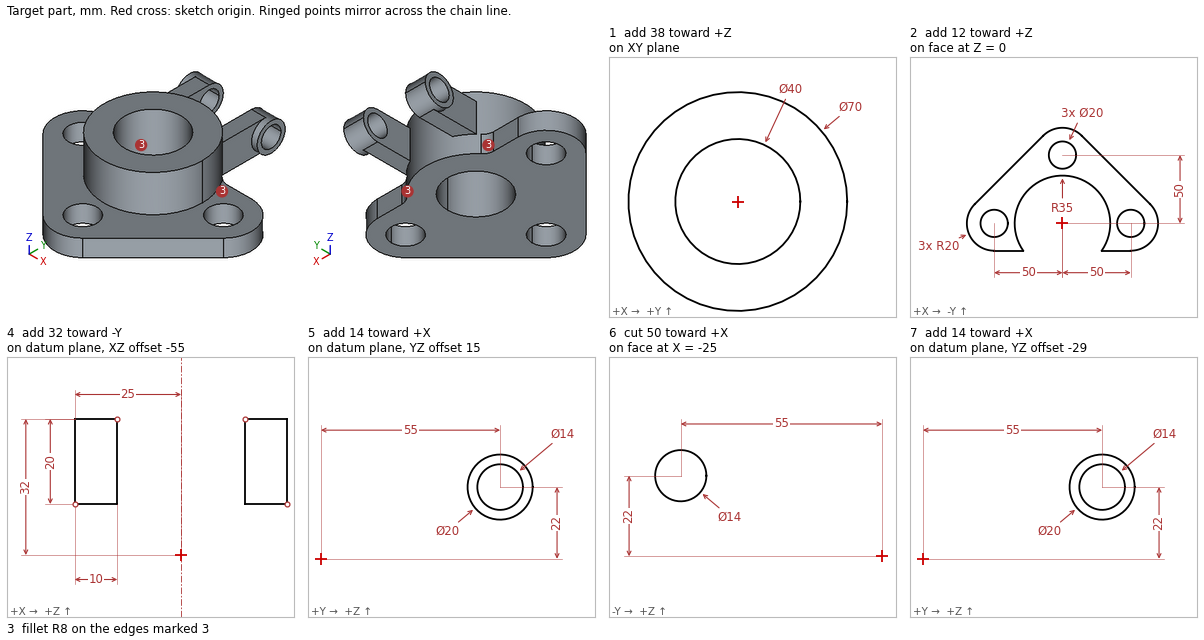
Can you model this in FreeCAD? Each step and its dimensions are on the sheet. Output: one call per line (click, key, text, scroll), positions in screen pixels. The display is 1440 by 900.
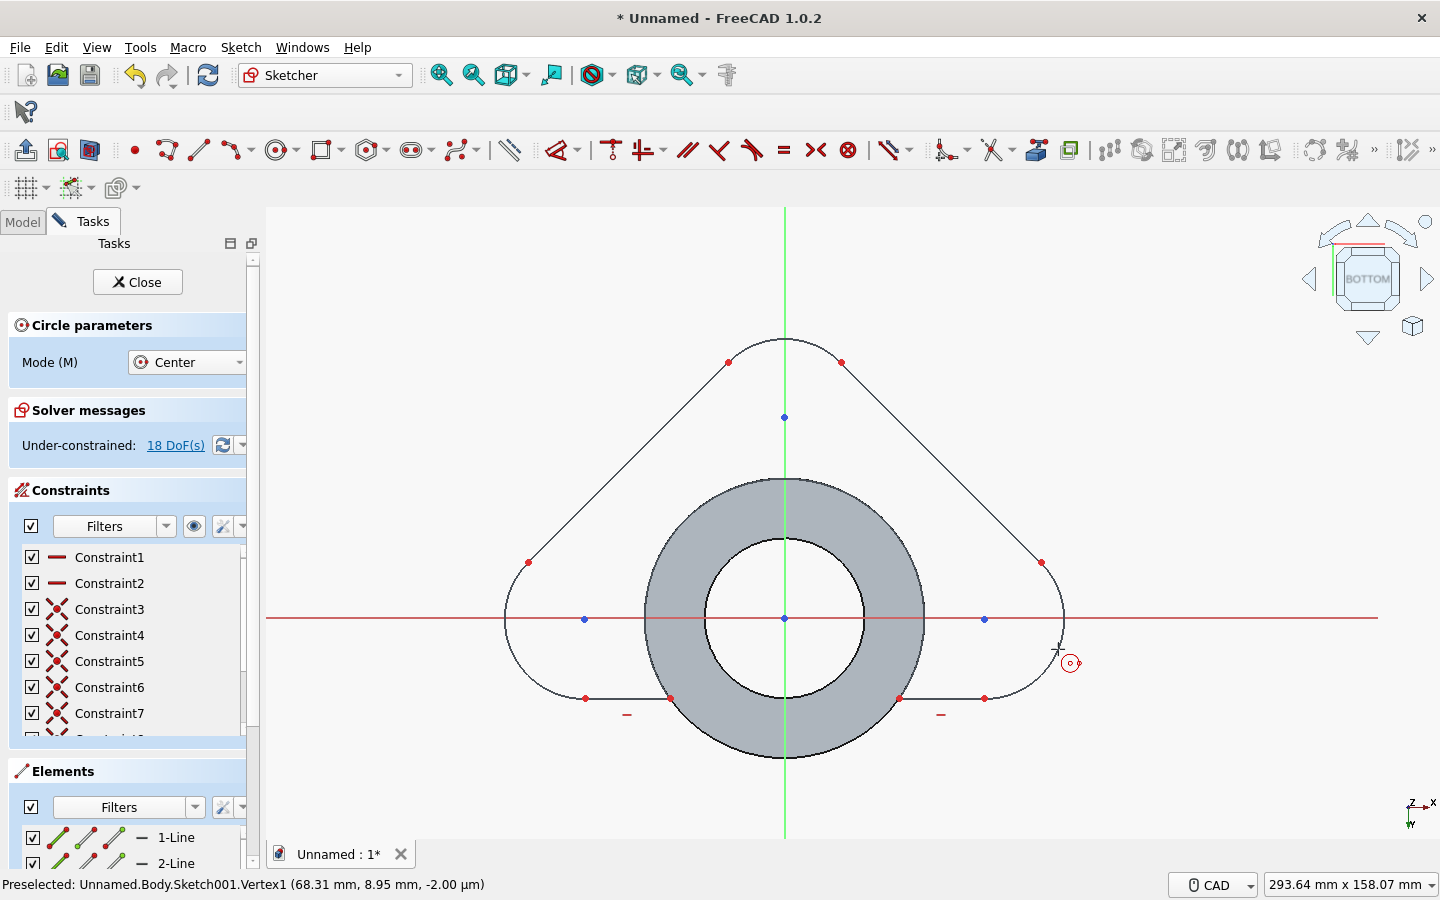
click(785, 418)
click(813, 390)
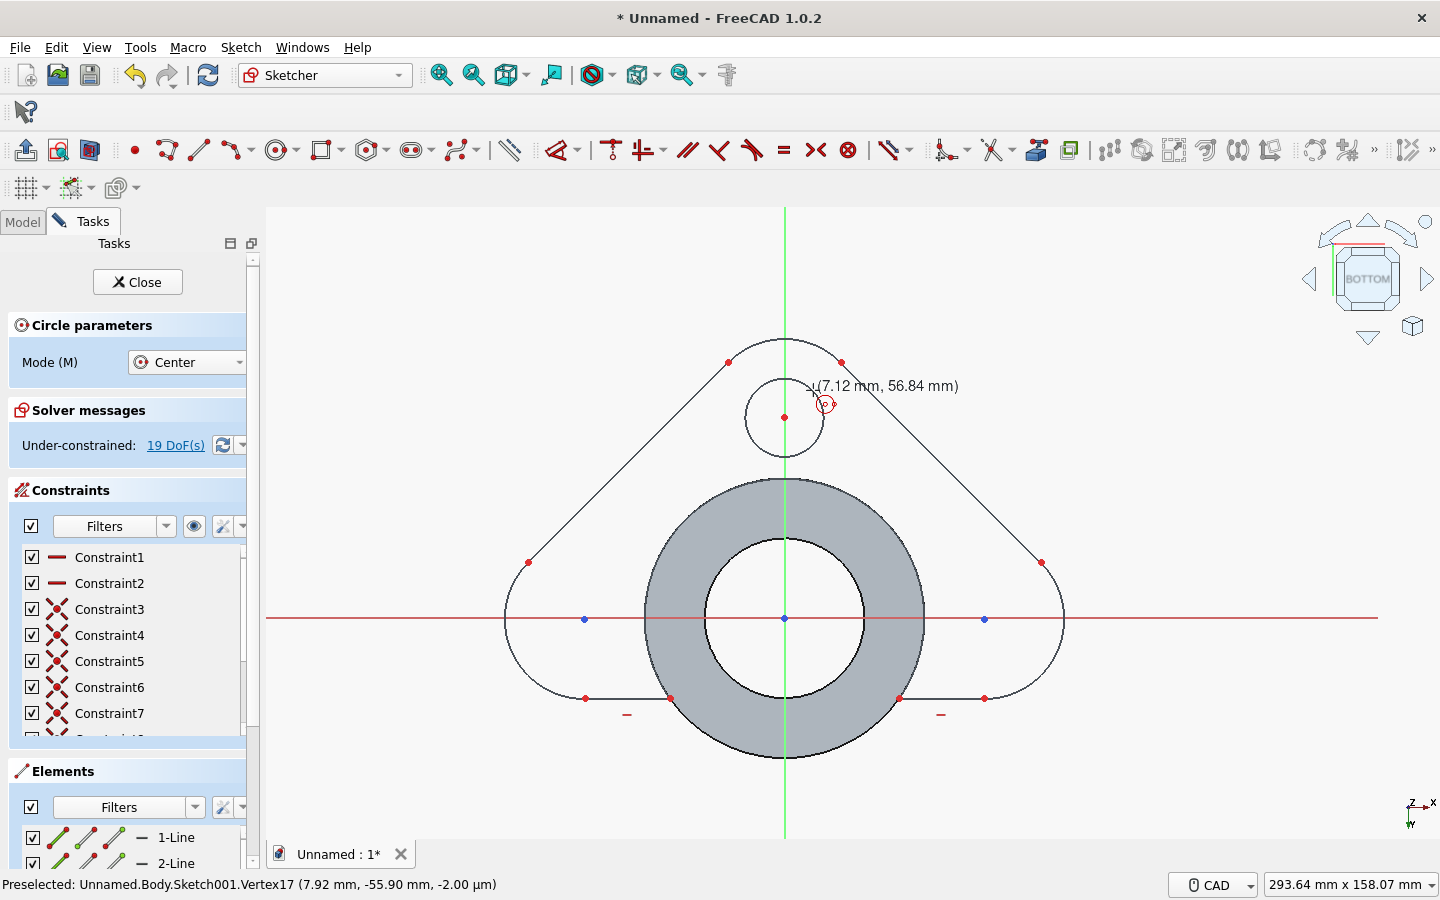
click(585, 618)
click(613, 590)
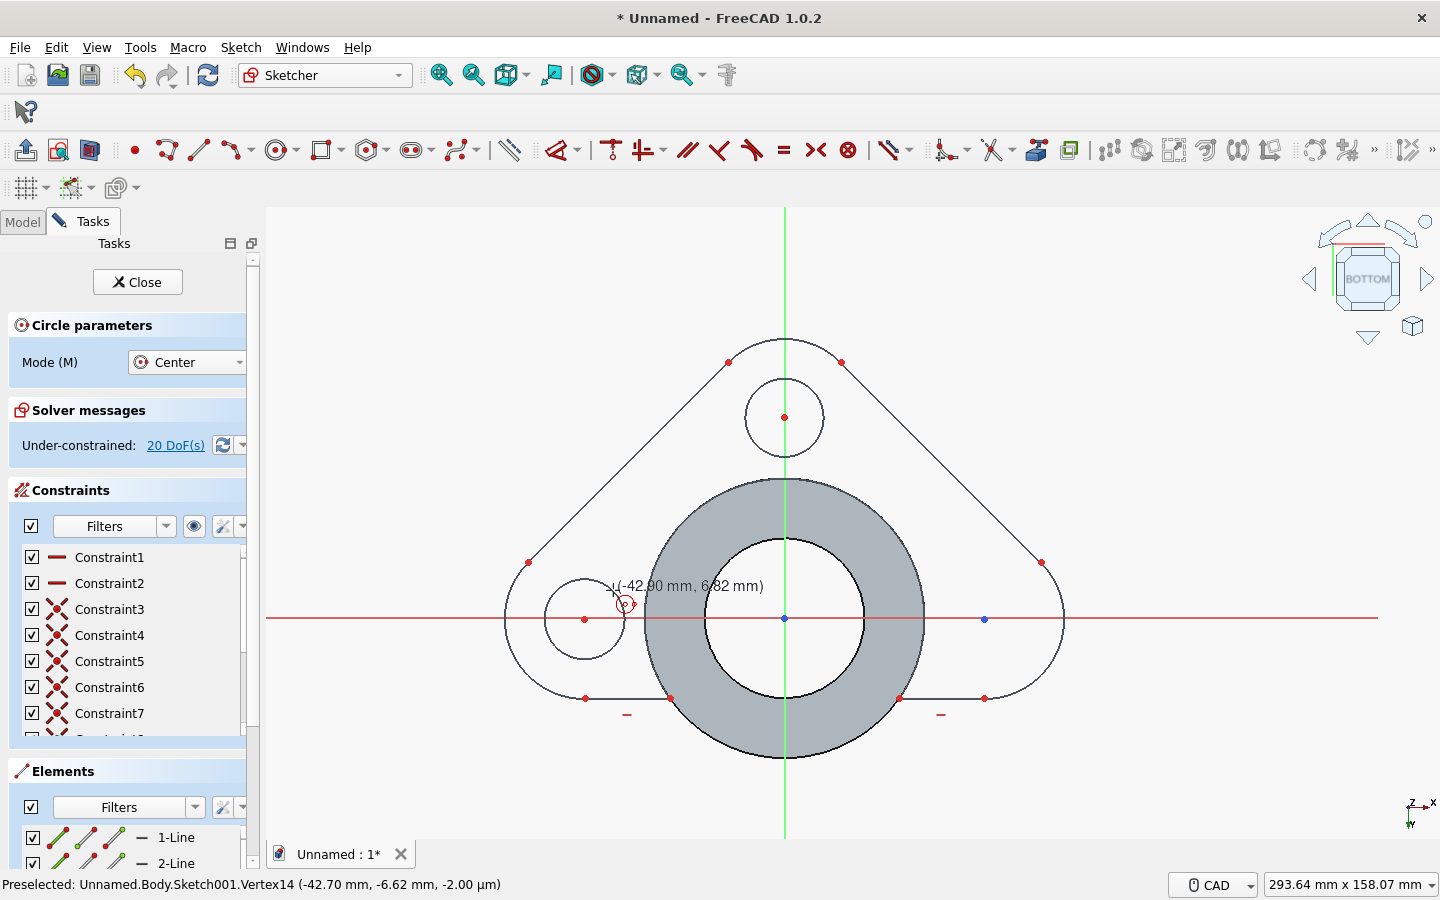
click(984, 618)
click(1013, 590)
key(Escape)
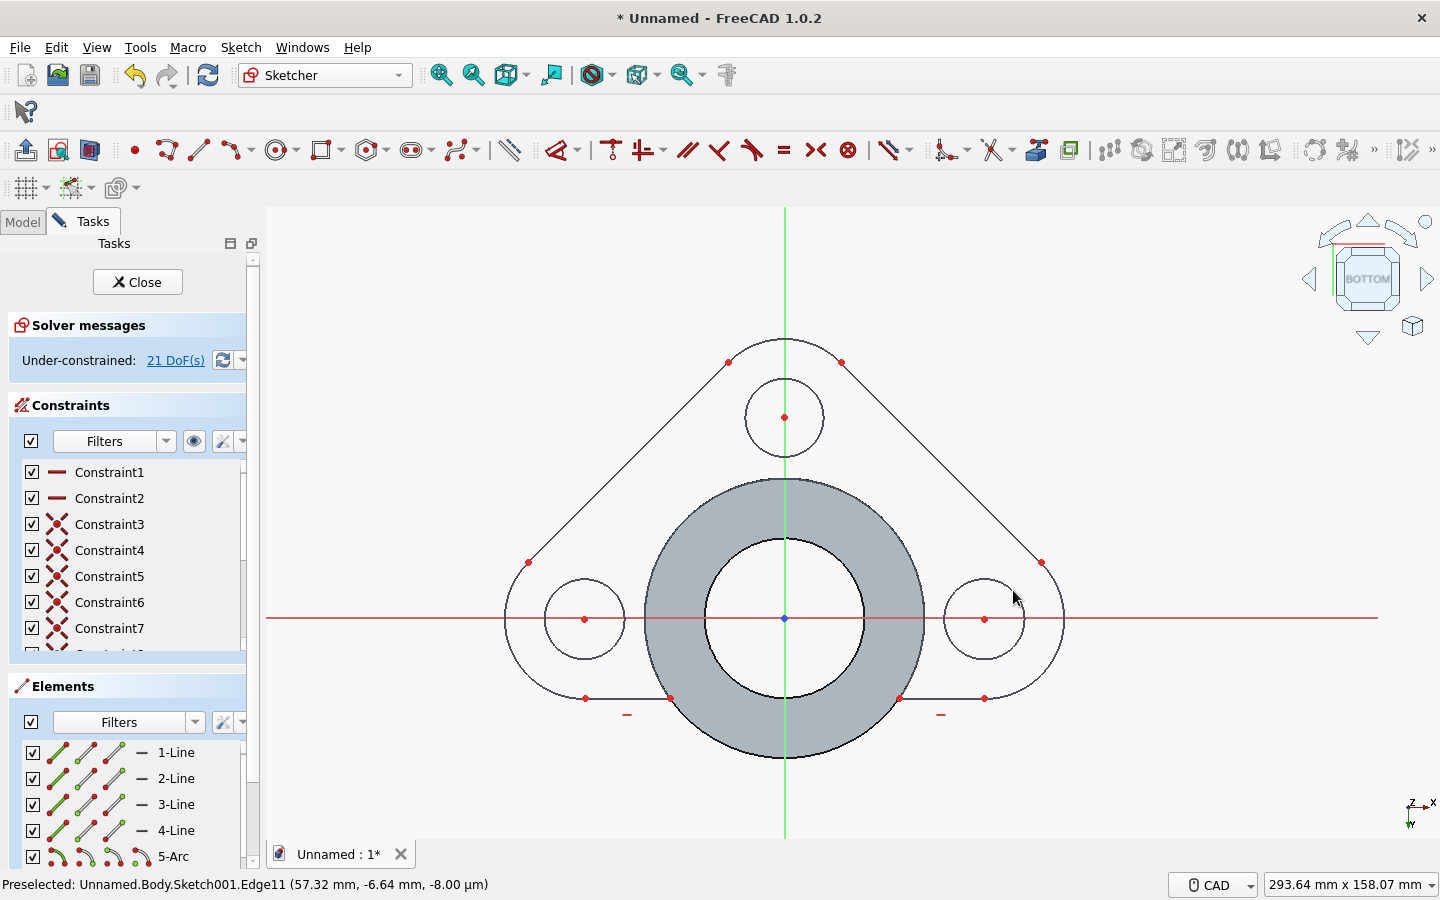
click(958, 699)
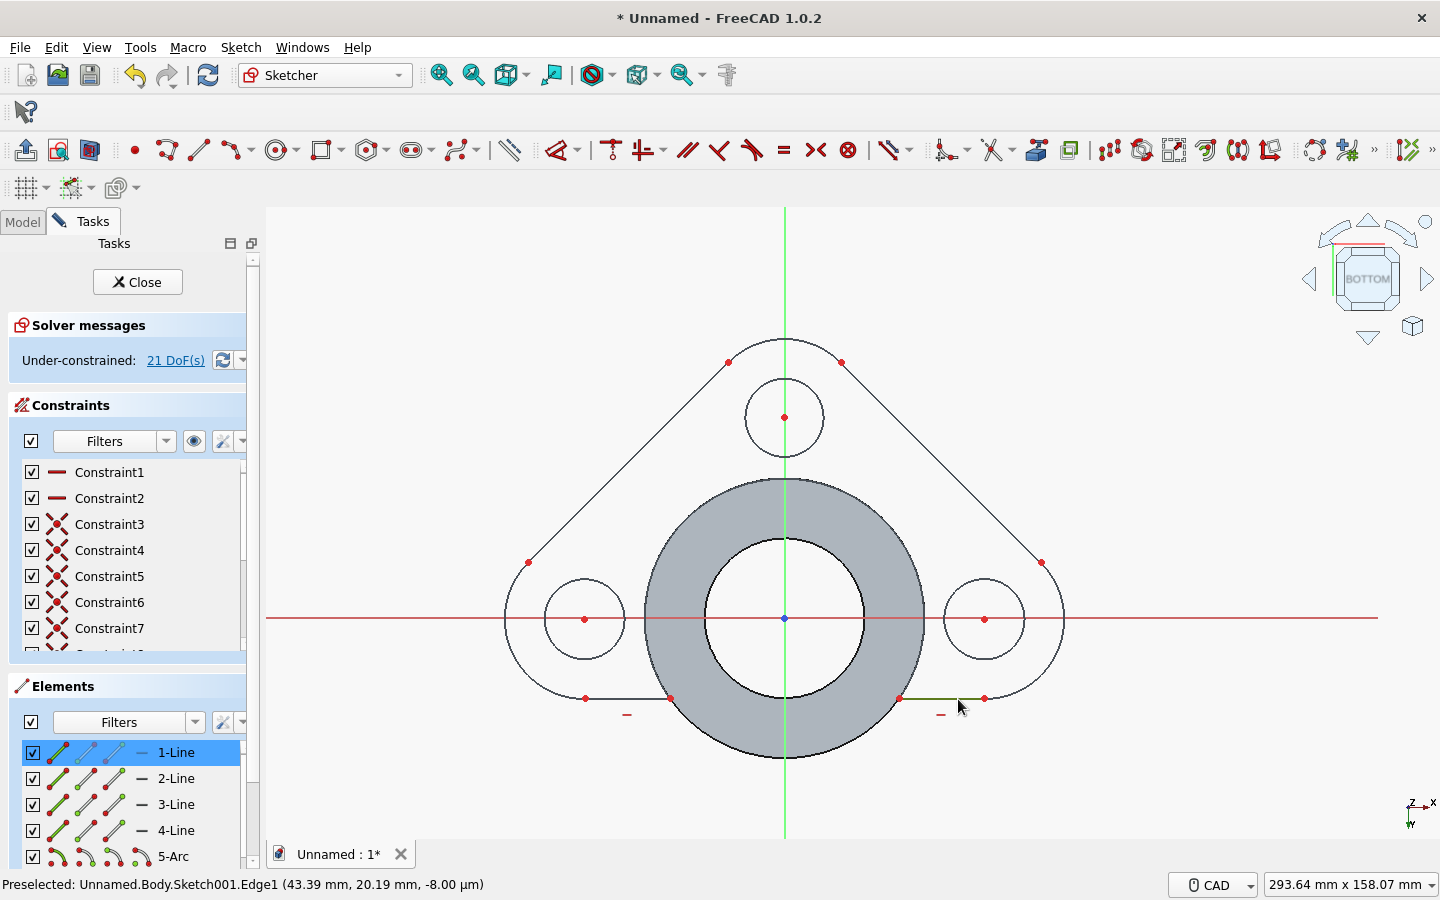
click(1036, 680)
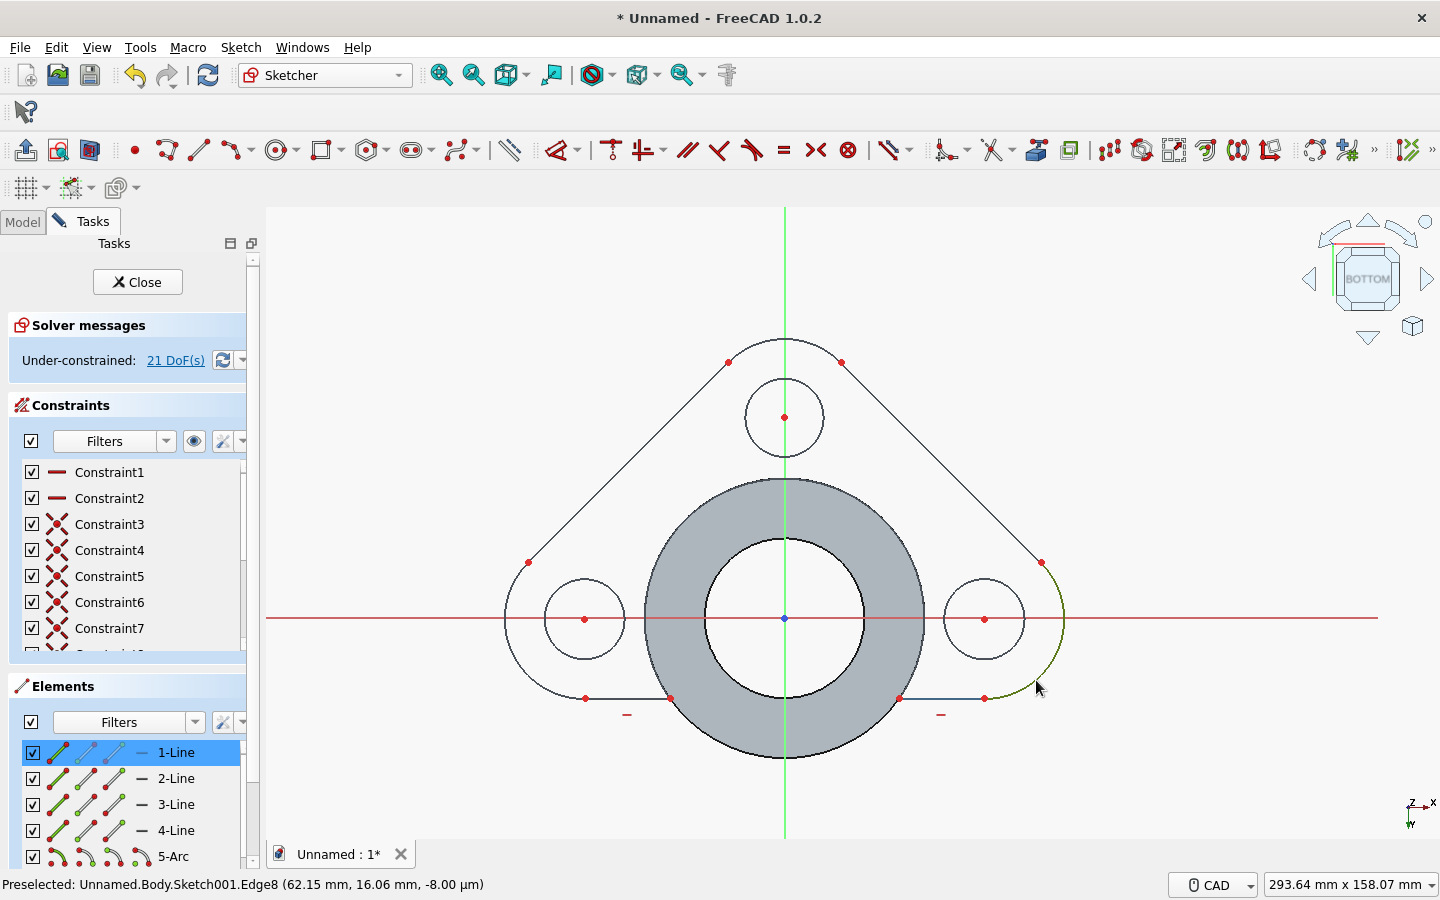
click(752, 150)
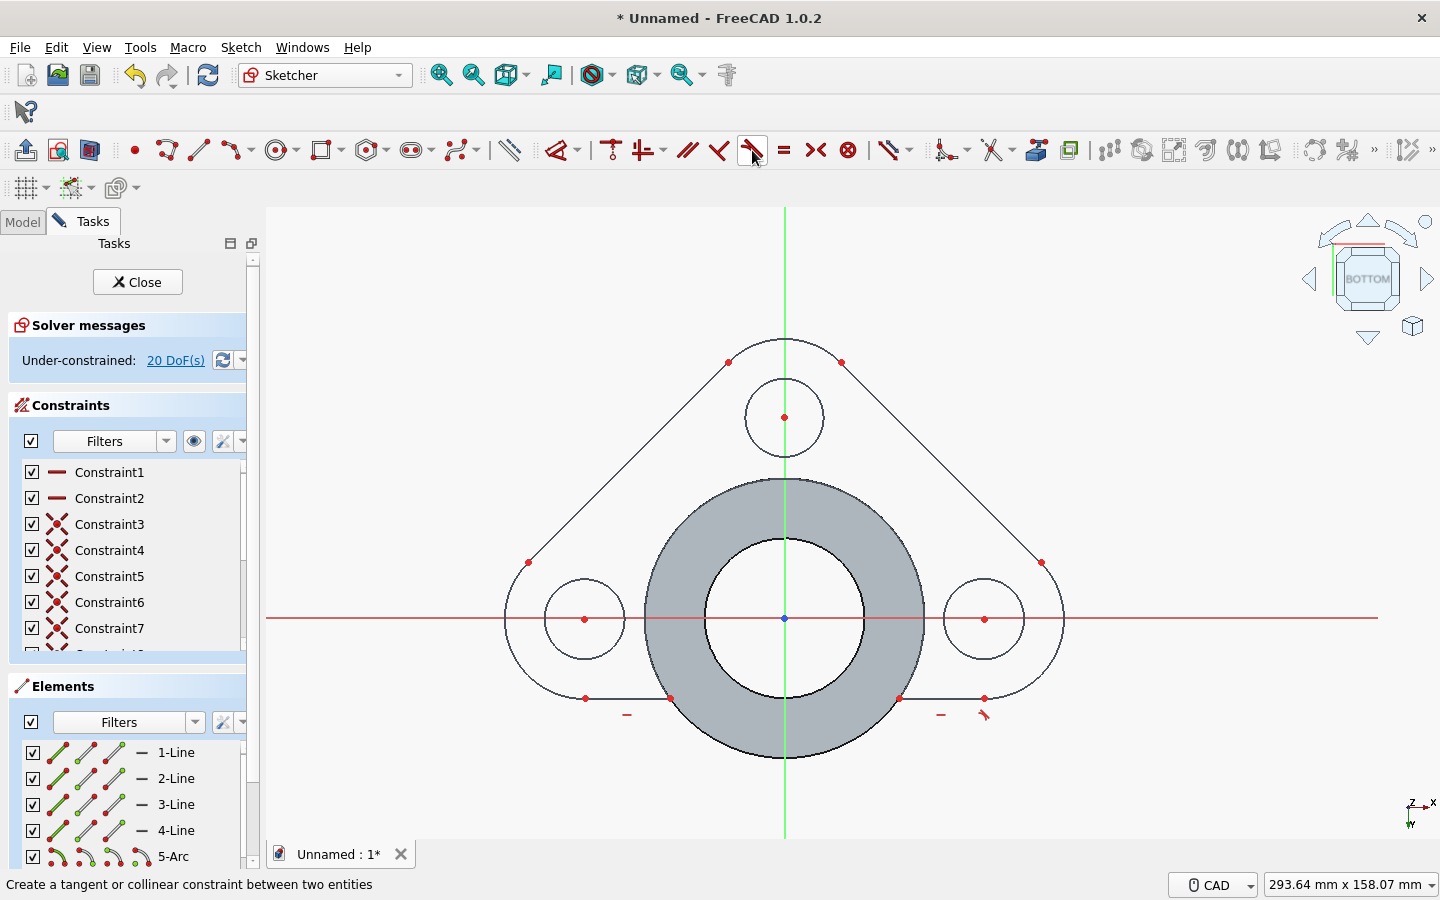
click(644, 699)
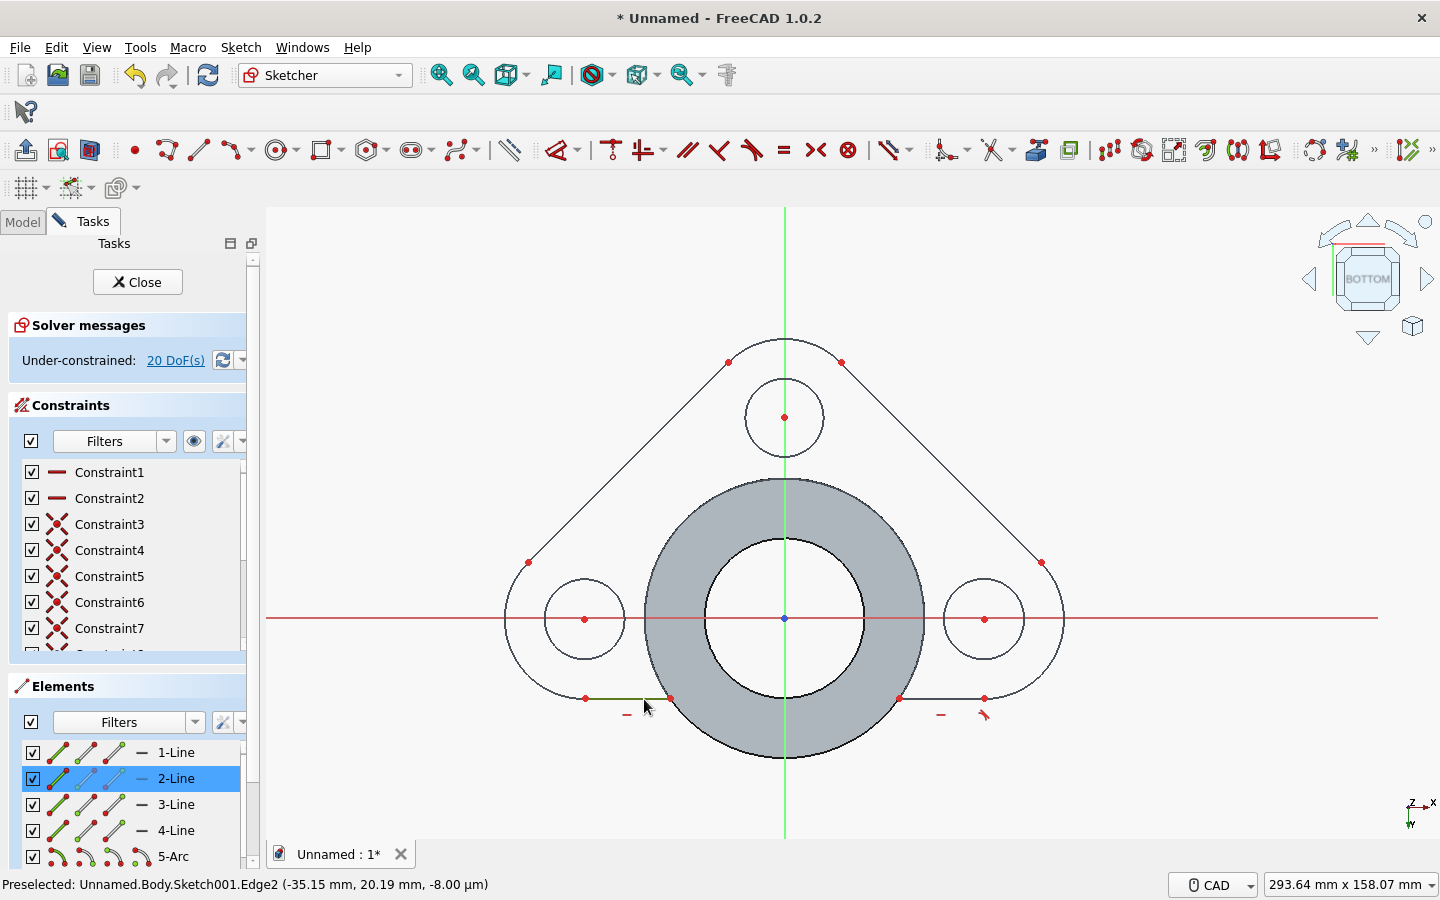
click(533, 680)